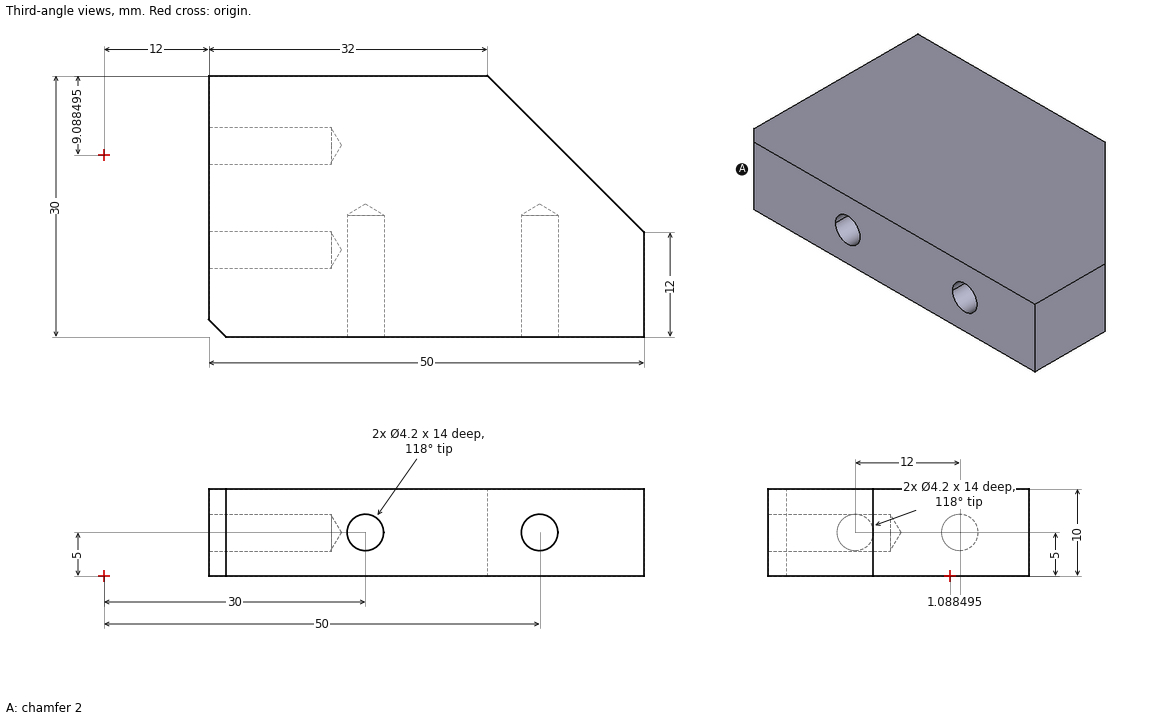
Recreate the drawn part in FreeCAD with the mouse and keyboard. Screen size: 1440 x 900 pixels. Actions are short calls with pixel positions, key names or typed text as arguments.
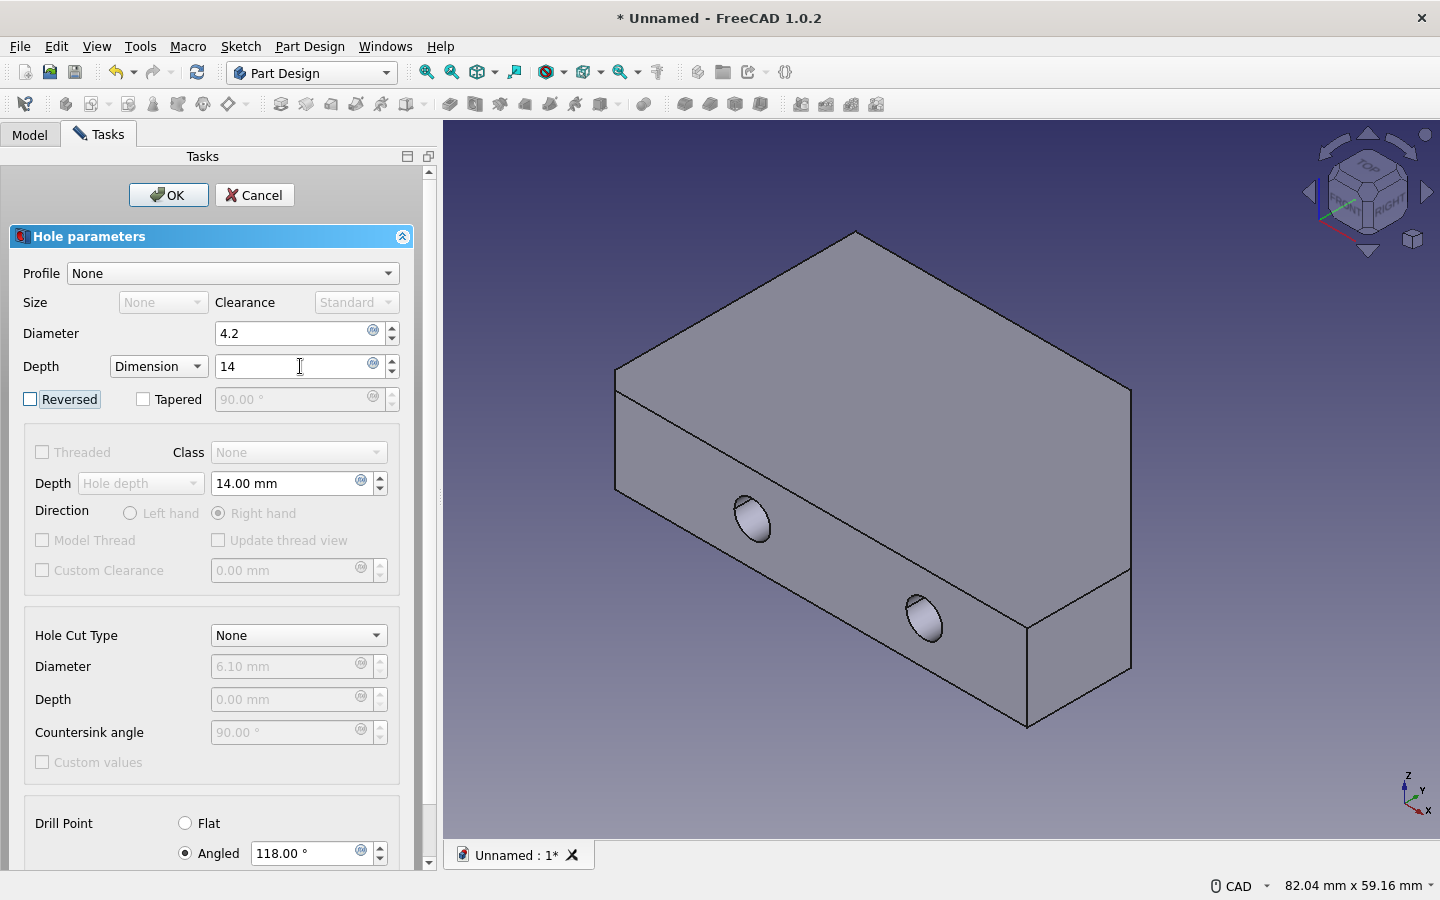
click(169, 195)